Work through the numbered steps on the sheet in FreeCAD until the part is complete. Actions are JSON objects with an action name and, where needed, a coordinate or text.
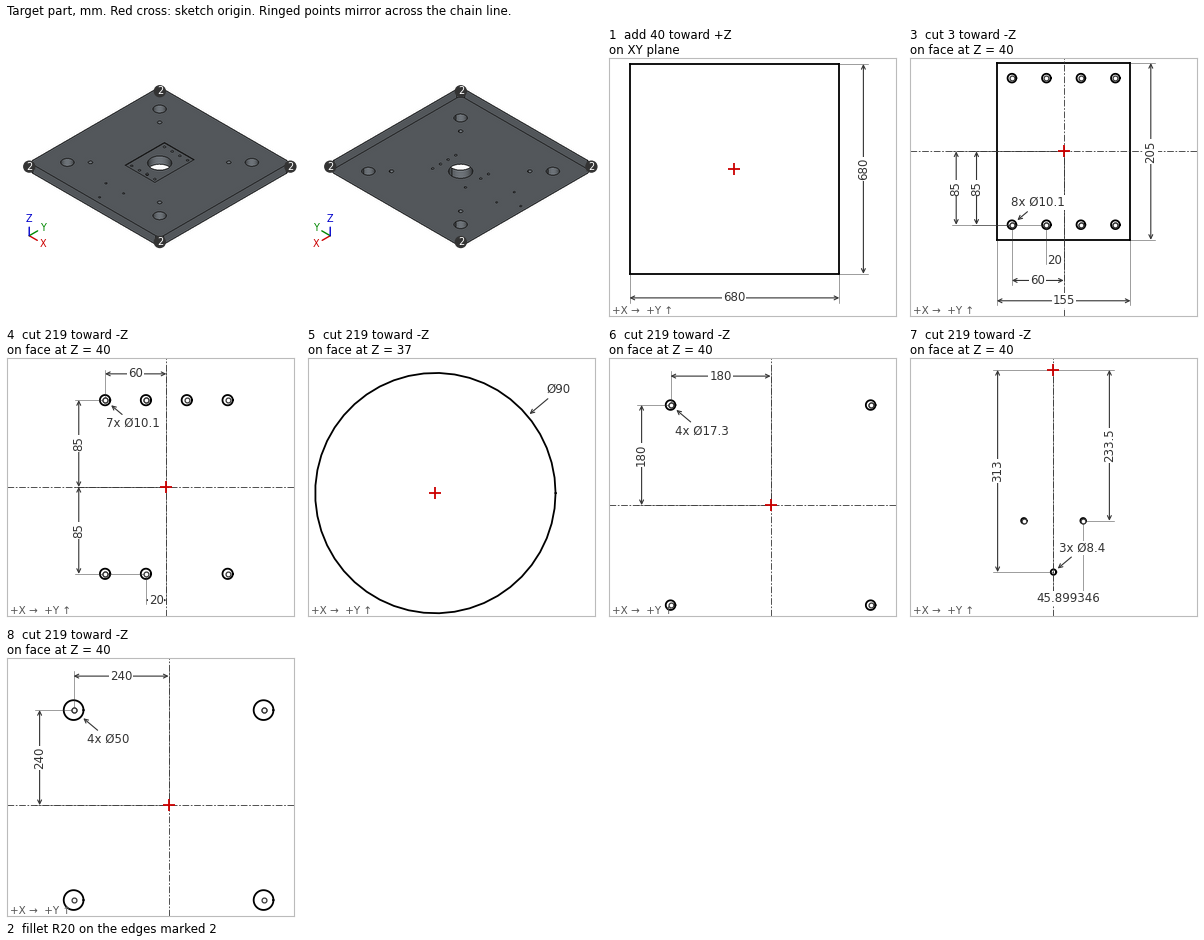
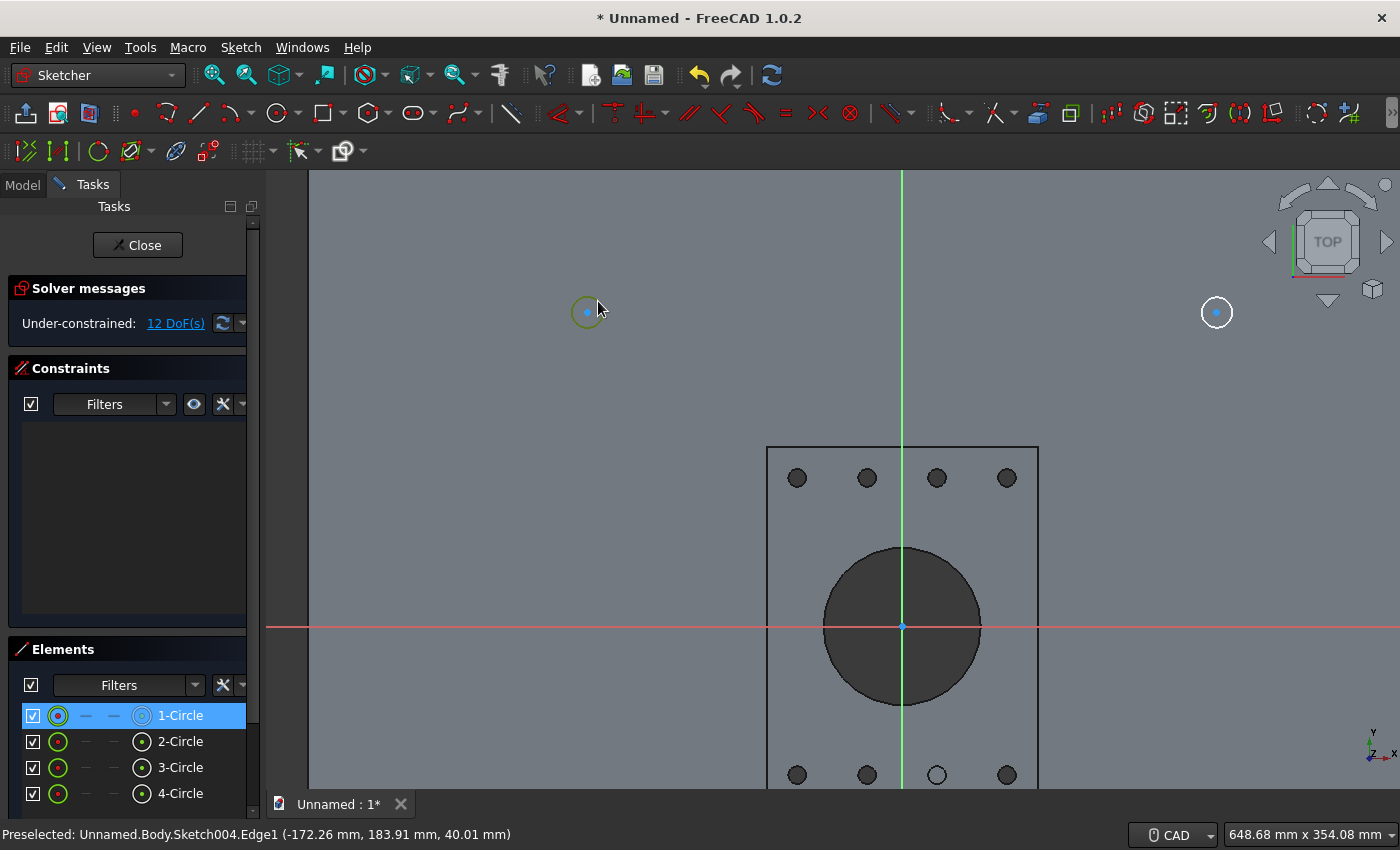
{"action": "left_click", "coordinate": [1228, 302]}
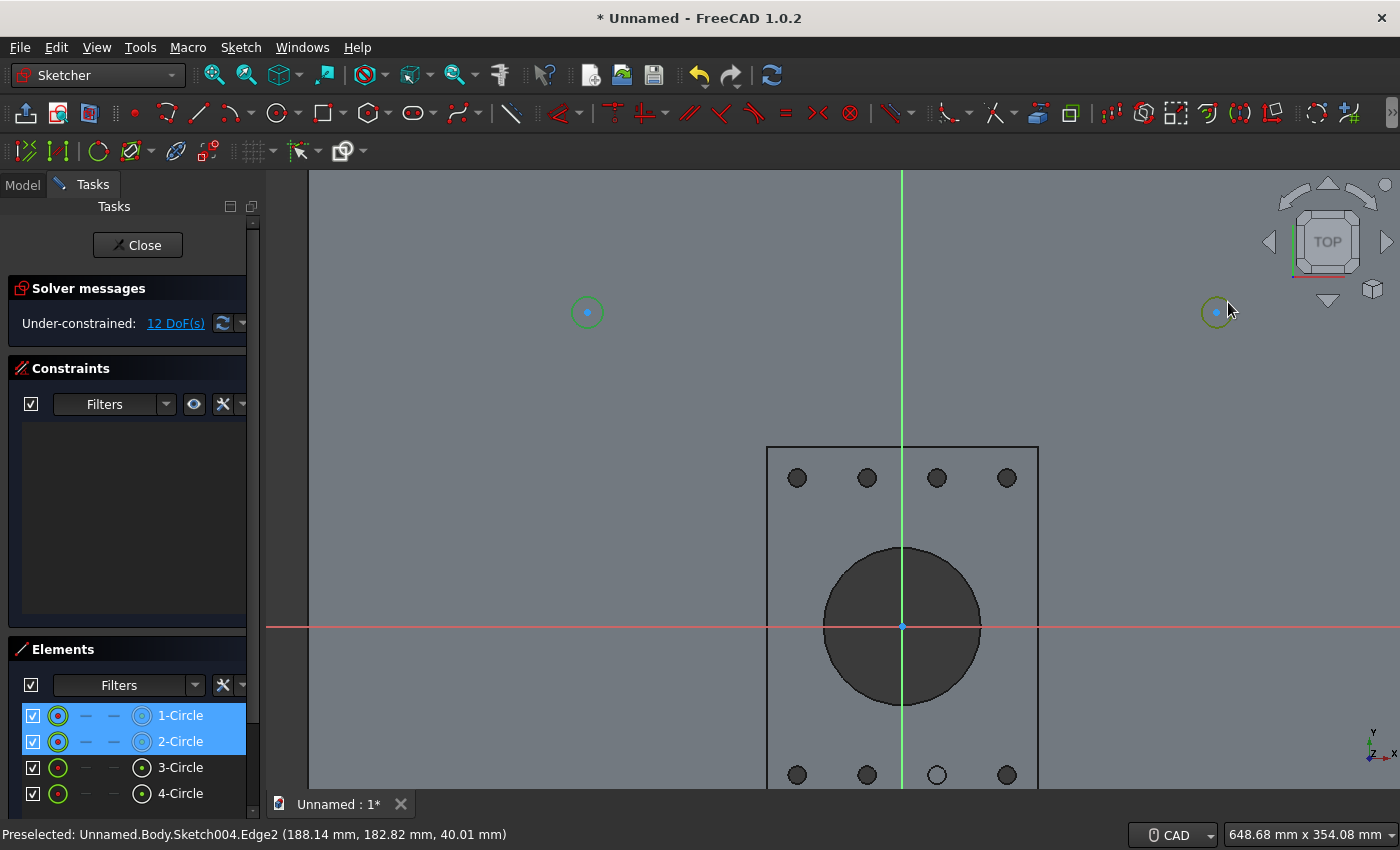
{"action": "scroll", "coordinate": [597, 301], "scroll_direction": "down", "scroll_amount": 3}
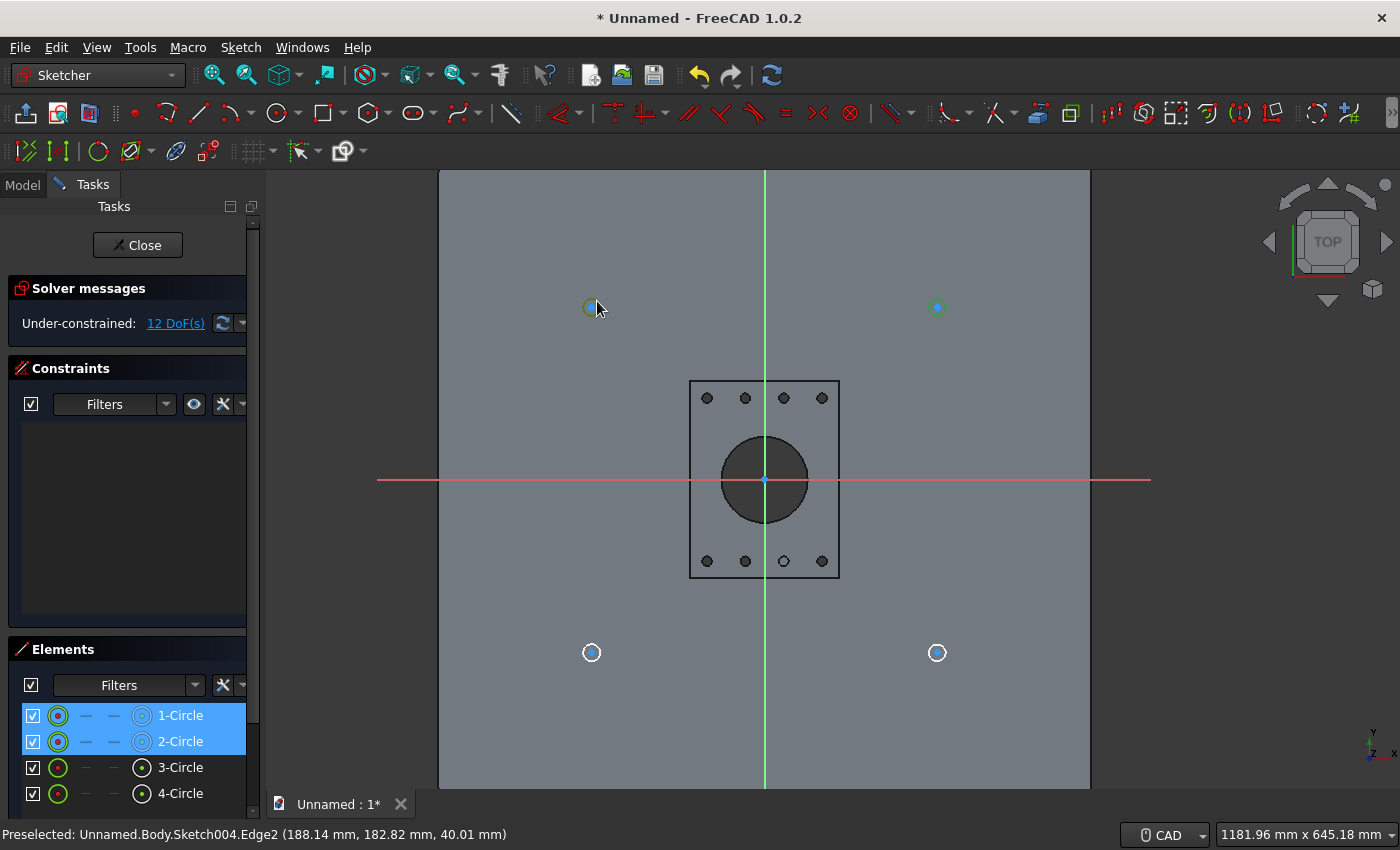
{"action": "scroll", "coordinate": [943, 647], "scroll_direction": "up", "scroll_amount": 3}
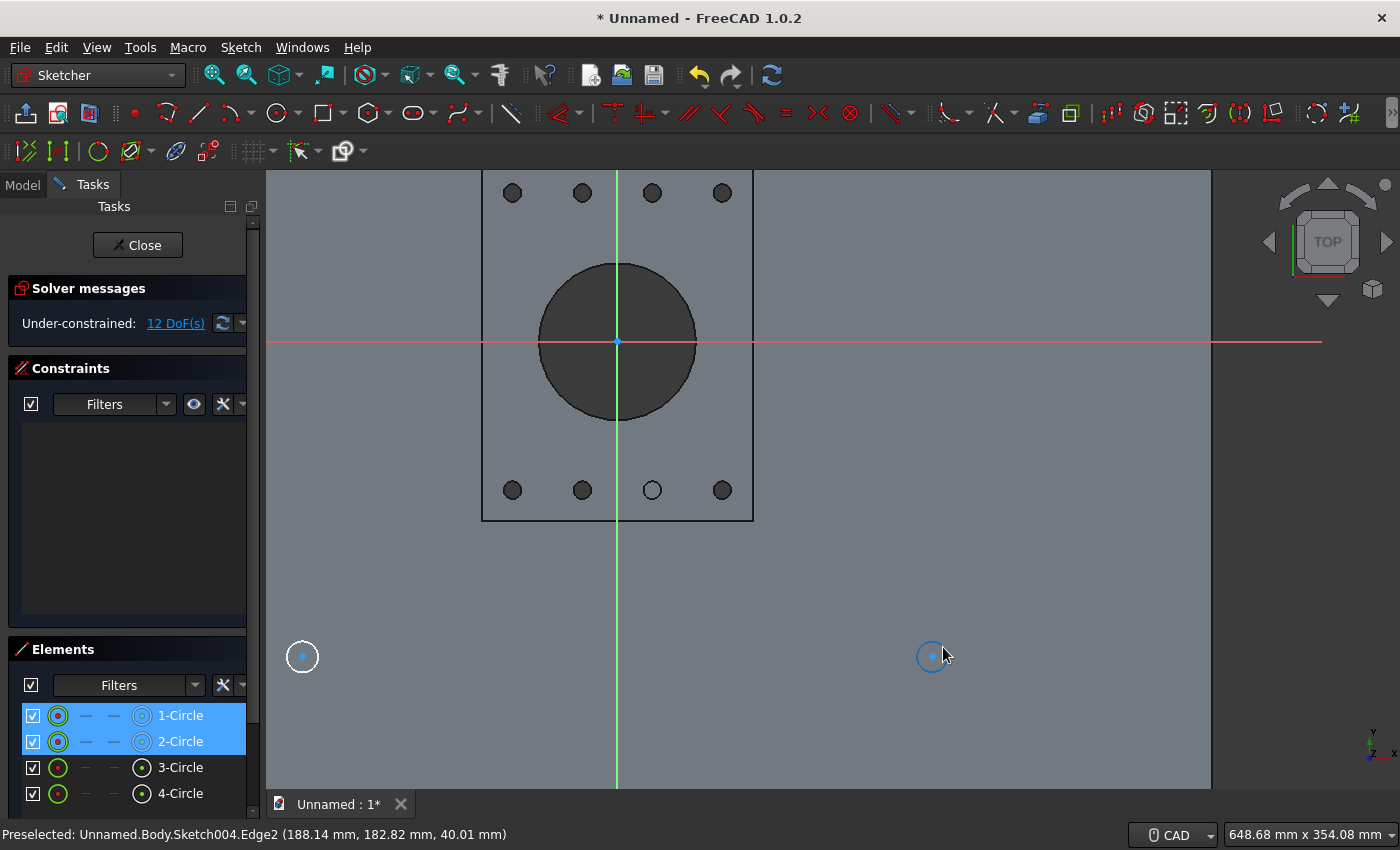
{"action": "left_click", "coordinate": [943, 646]}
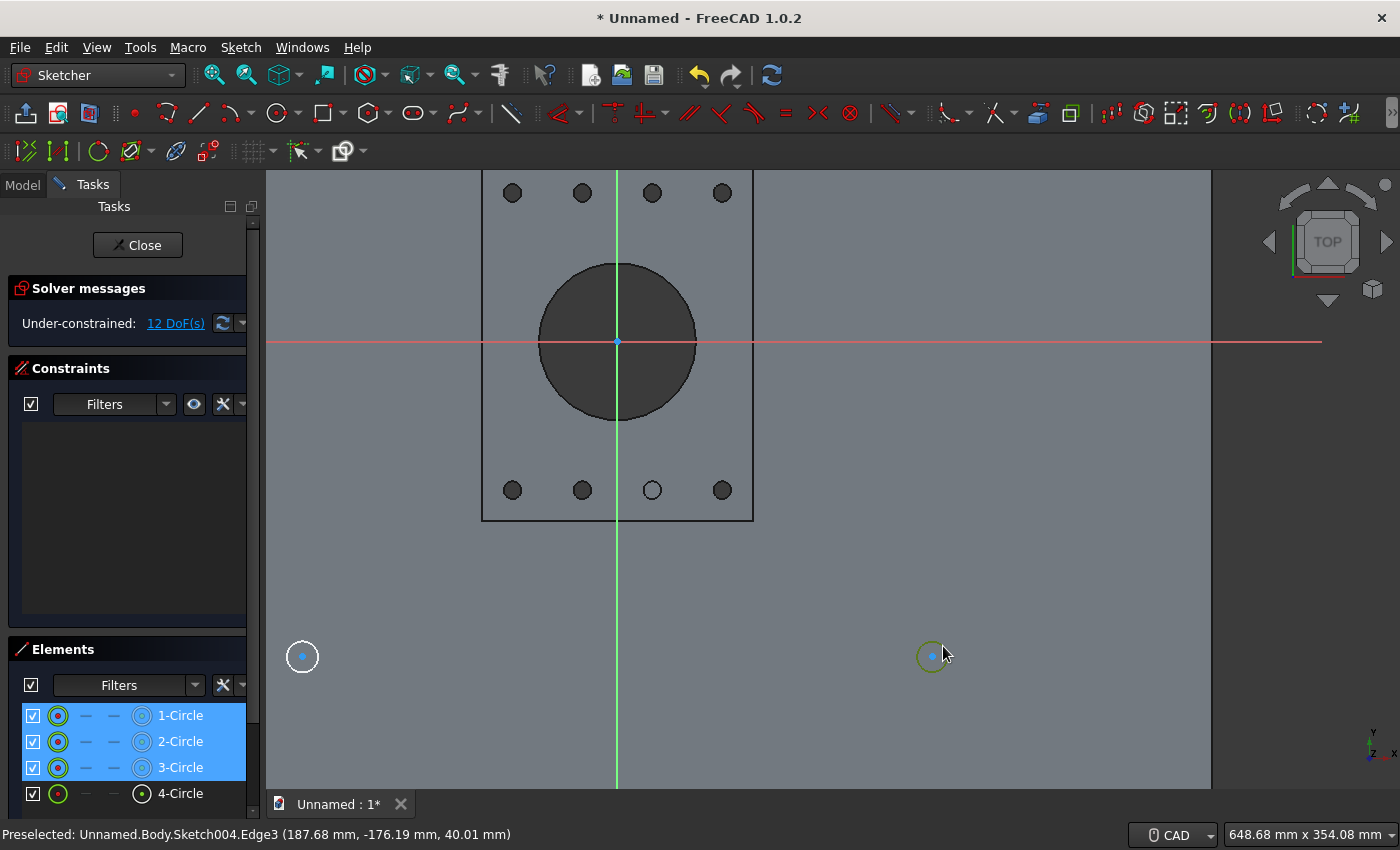
{"action": "left_click", "coordinate": [313, 646]}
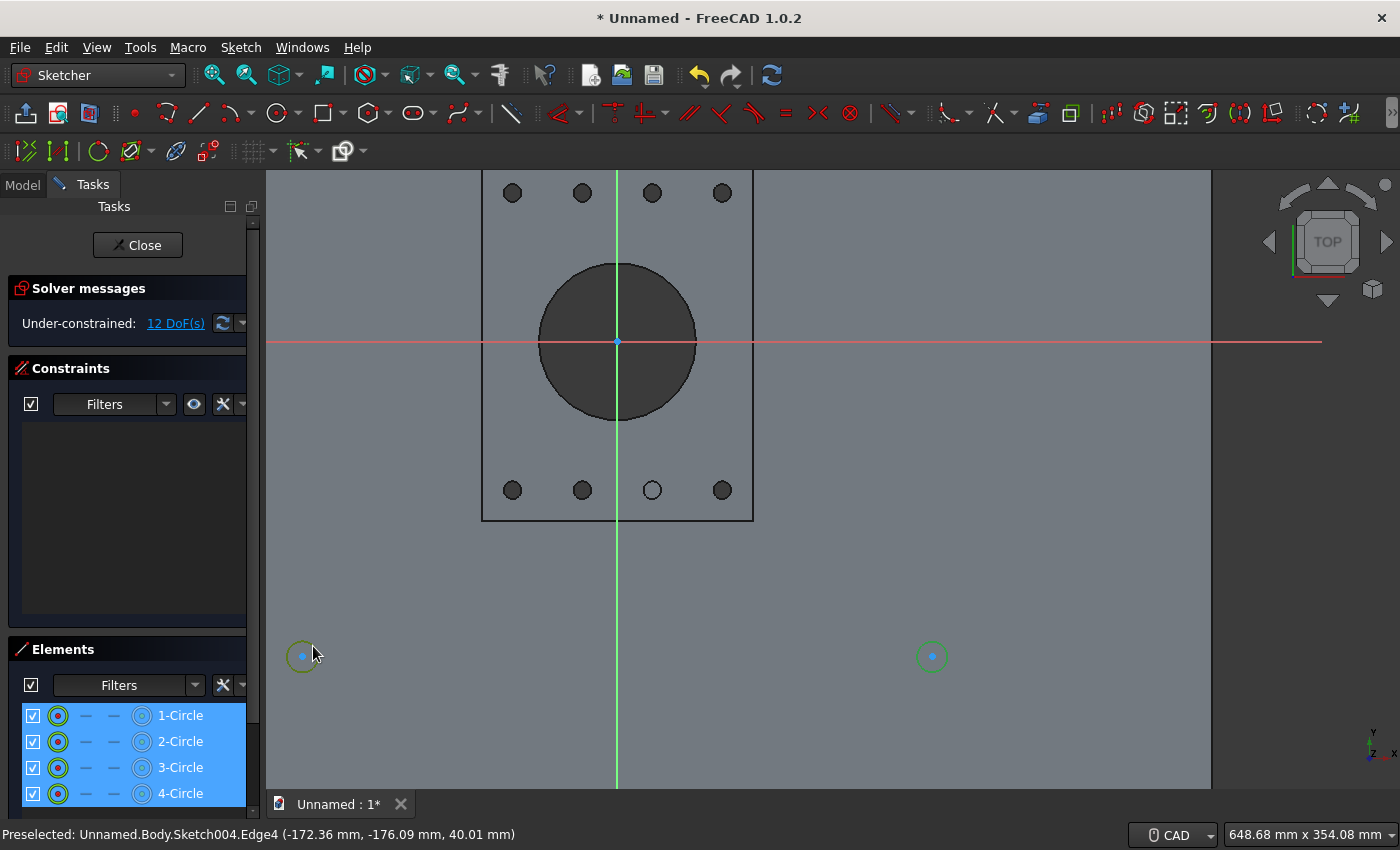
{"action": "left_click", "coordinate": [786, 114]}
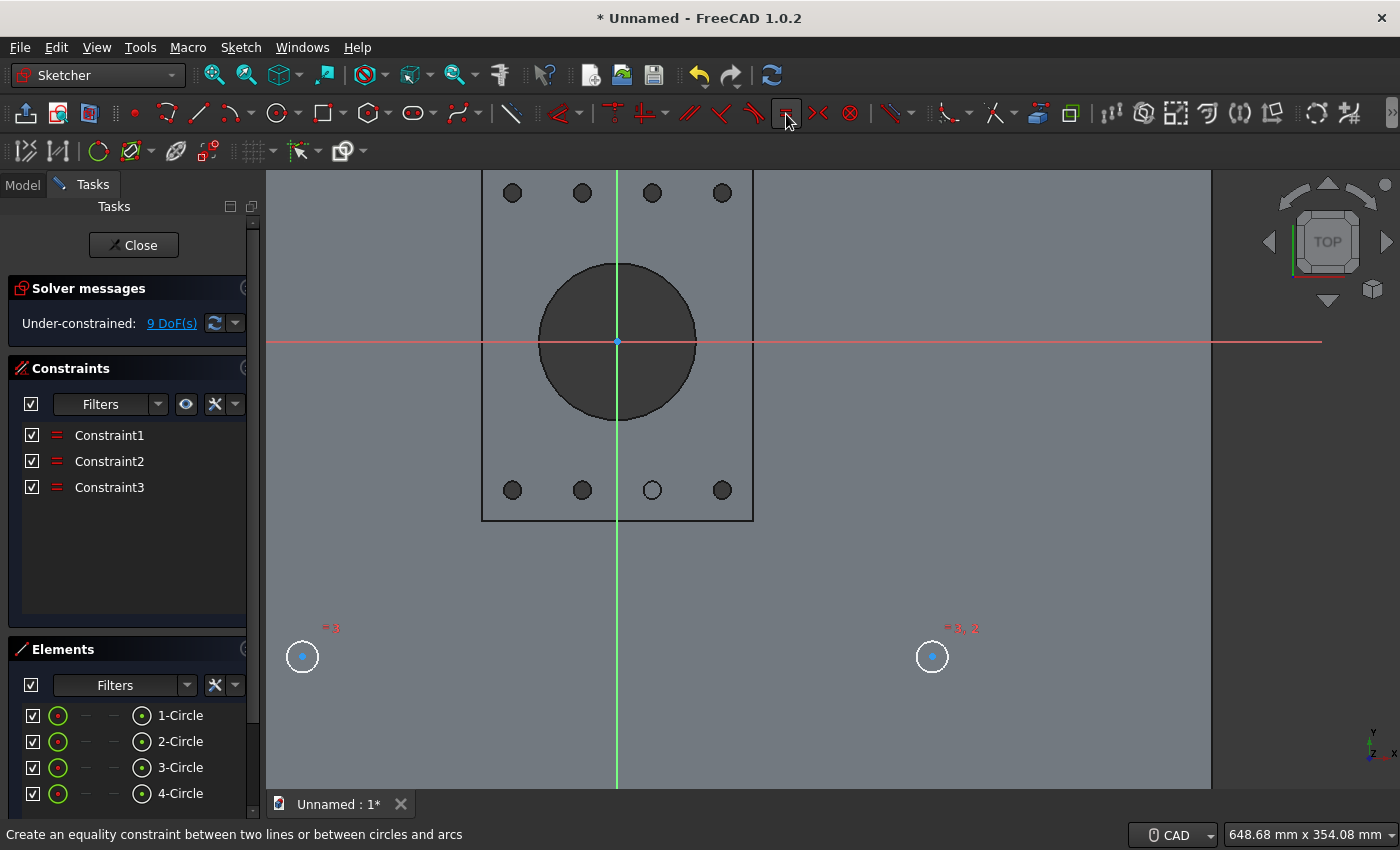
{"action": "scroll", "coordinate": [943, 647], "scroll_direction": "down", "scroll_amount": 3}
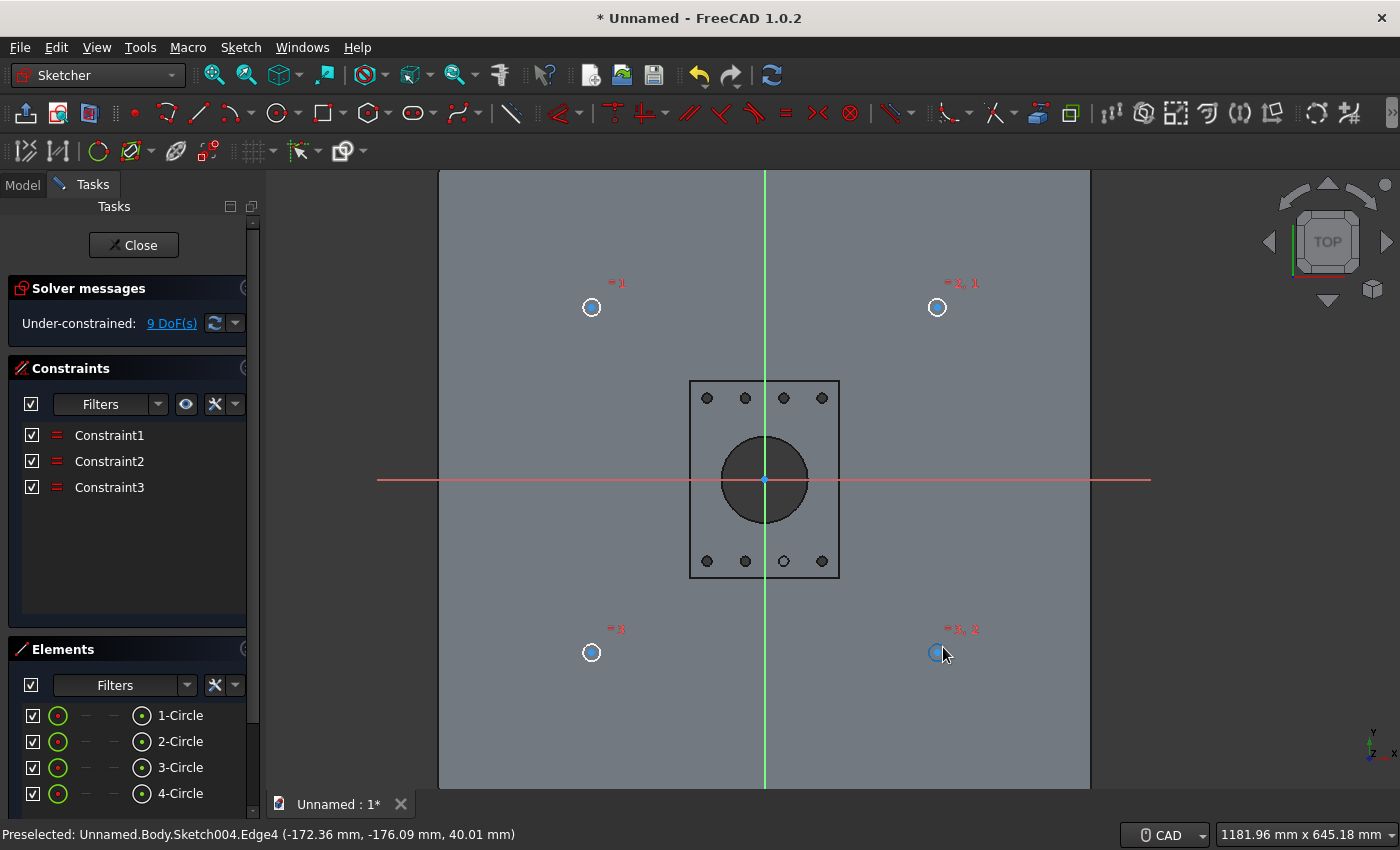
{"action": "left_click", "coordinate": [592, 307]}